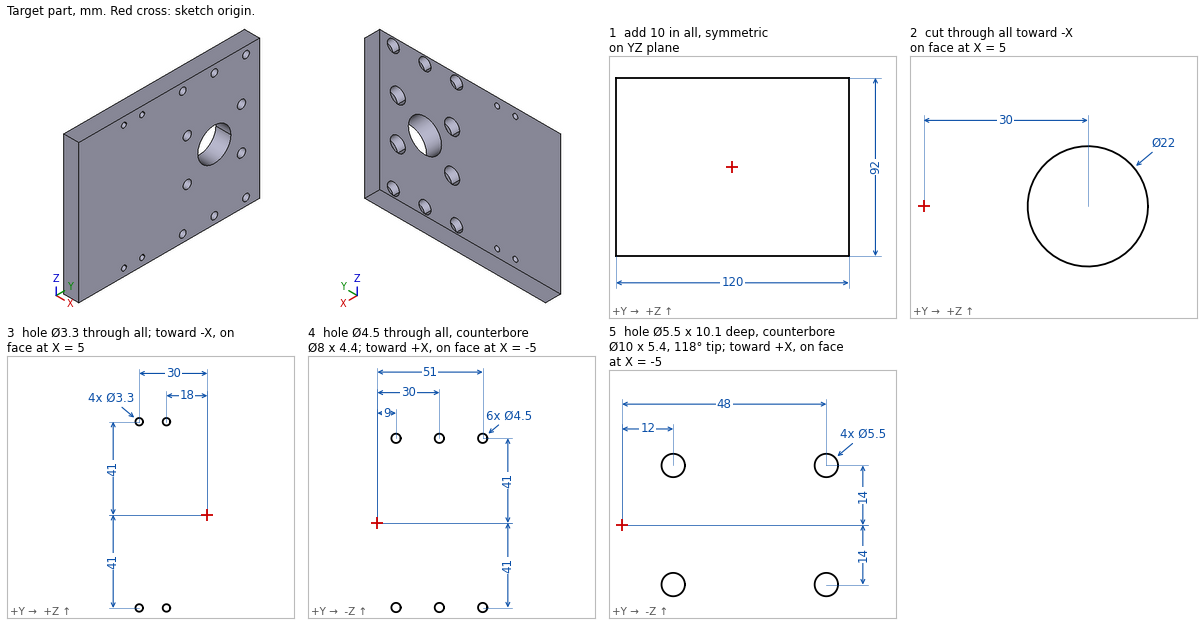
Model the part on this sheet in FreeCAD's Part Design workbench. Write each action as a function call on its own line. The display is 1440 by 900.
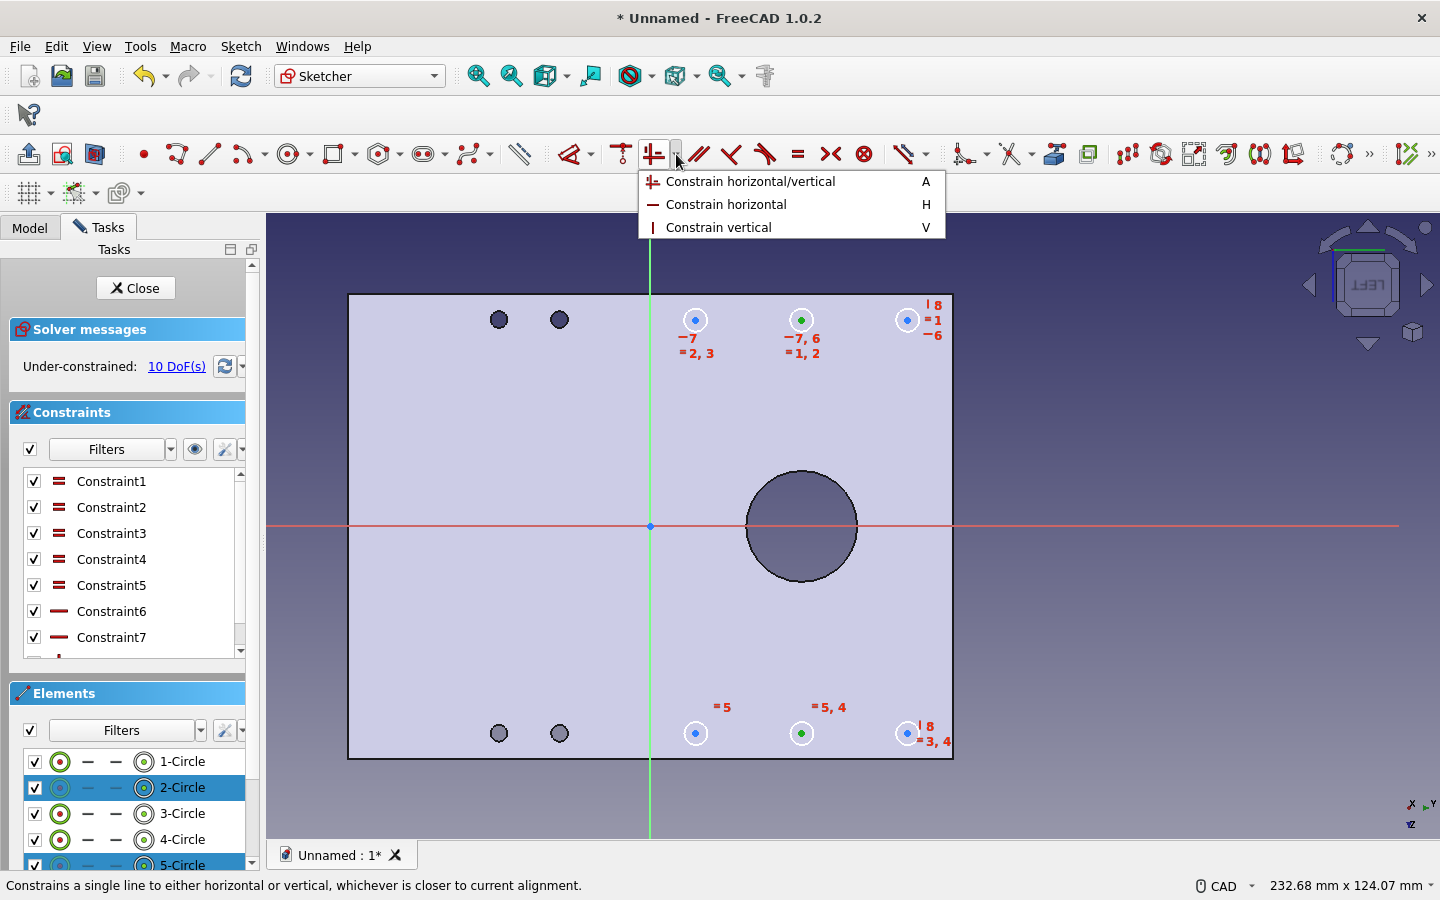
click(792, 228)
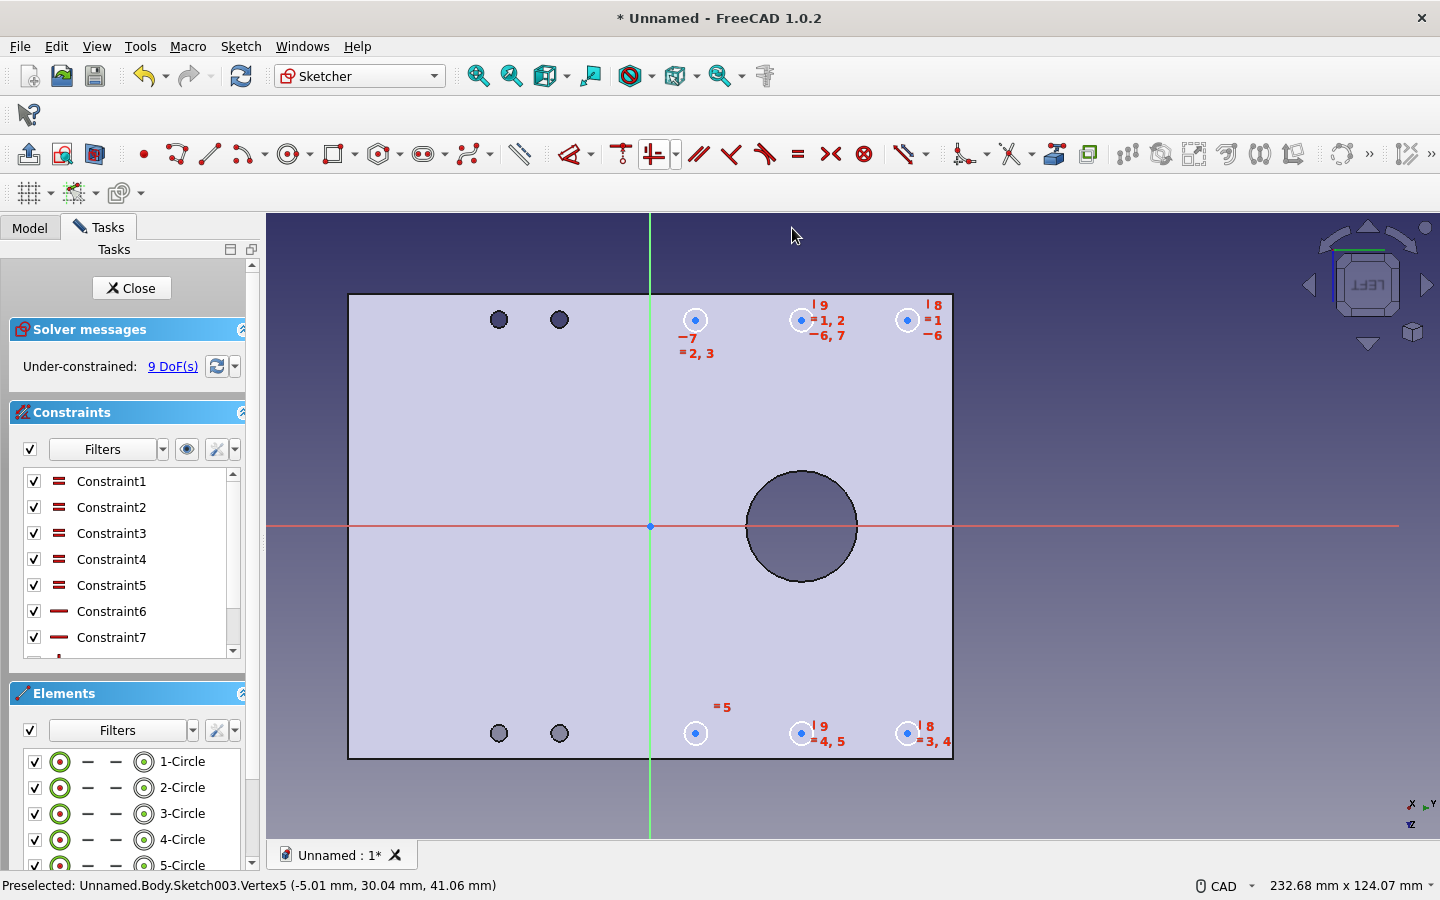
click(908, 734)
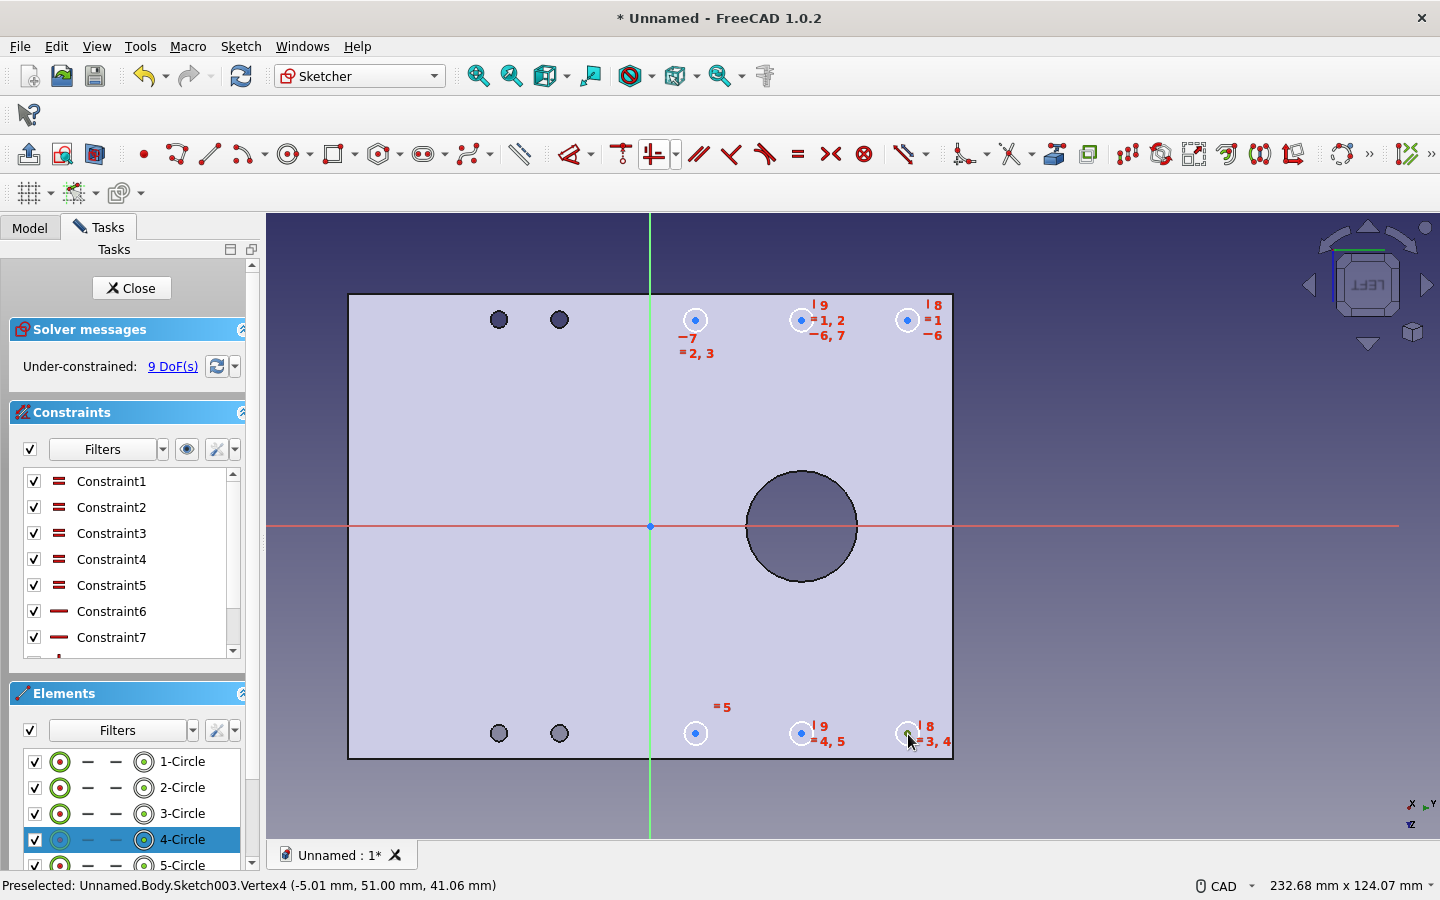
click(802, 734)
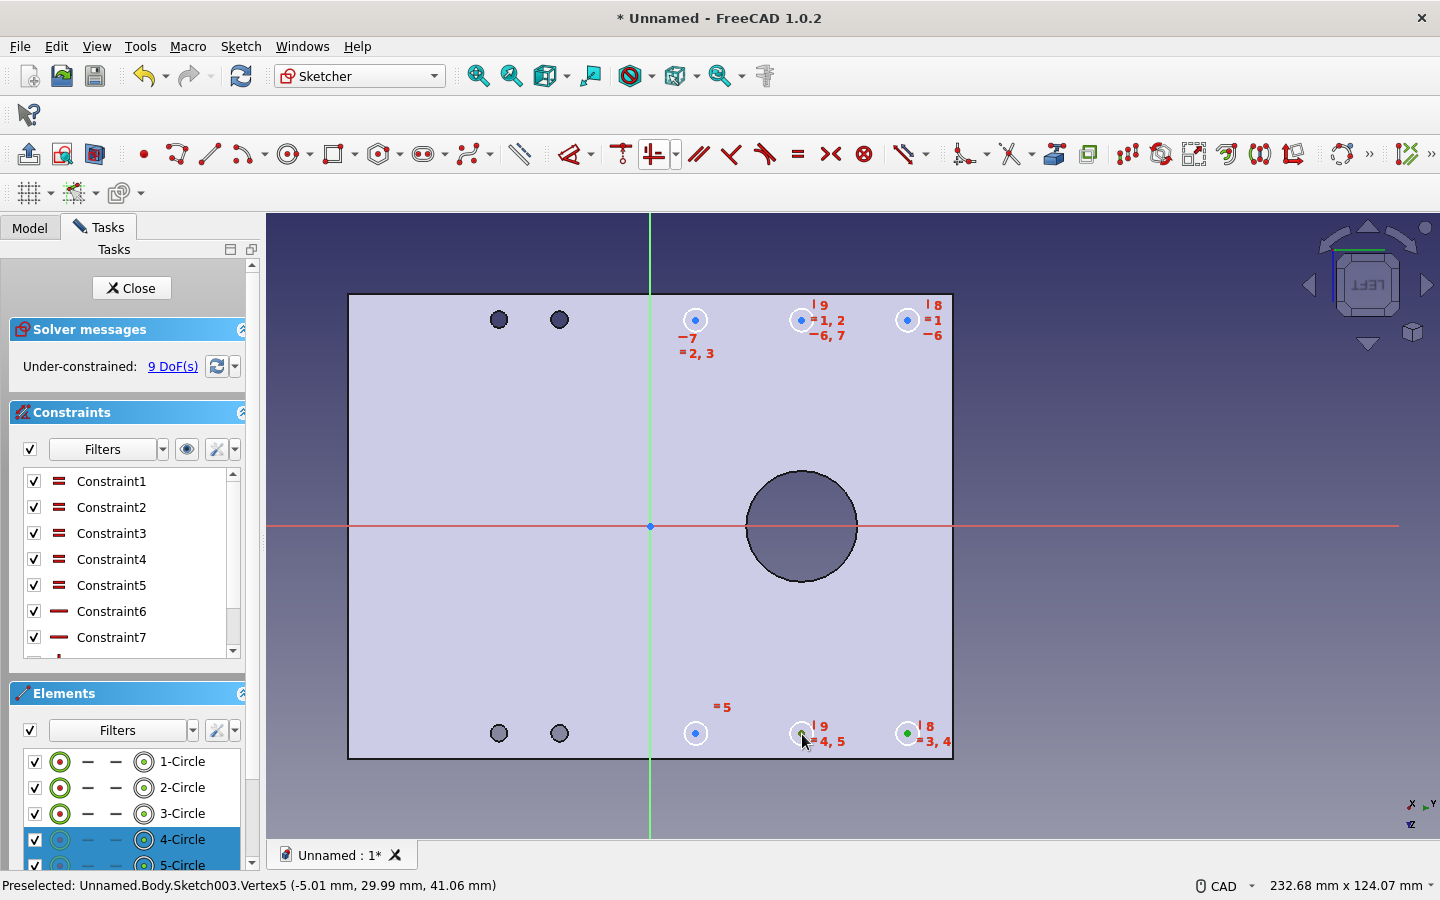
key(h)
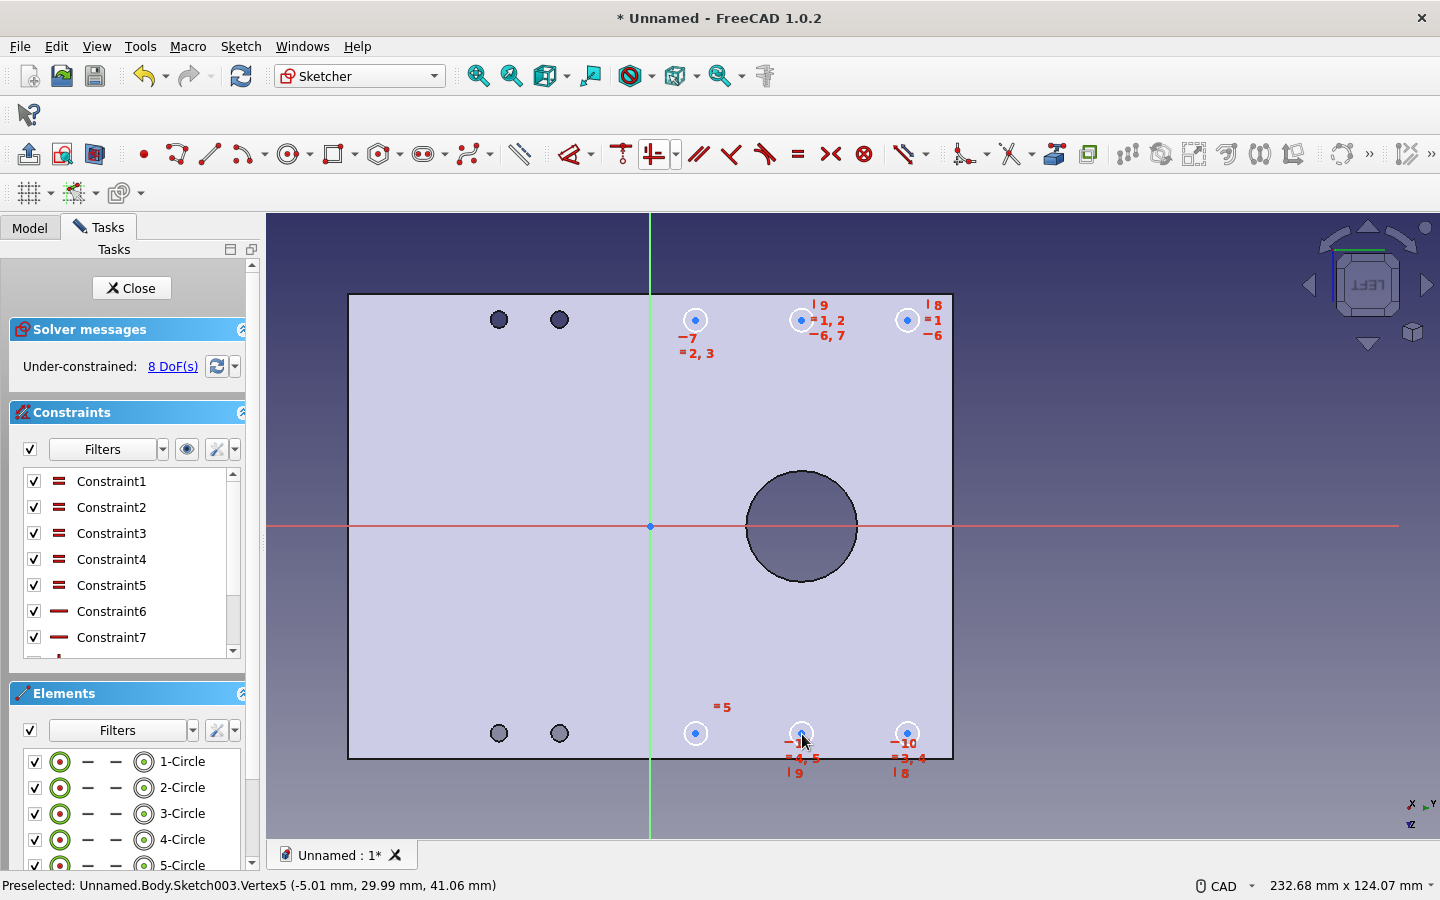
click(696, 320)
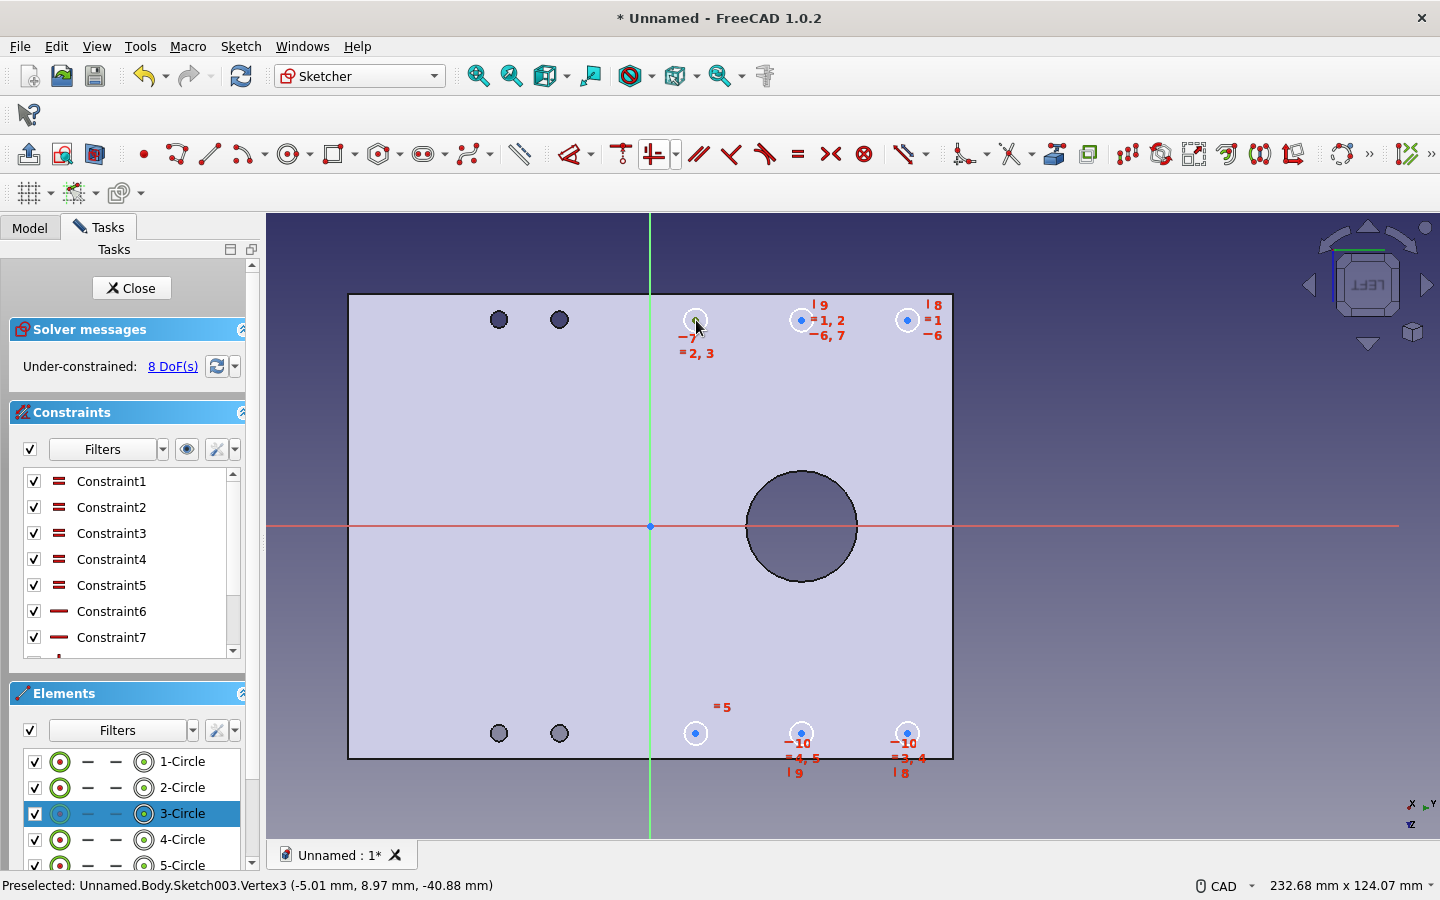
click(696, 734)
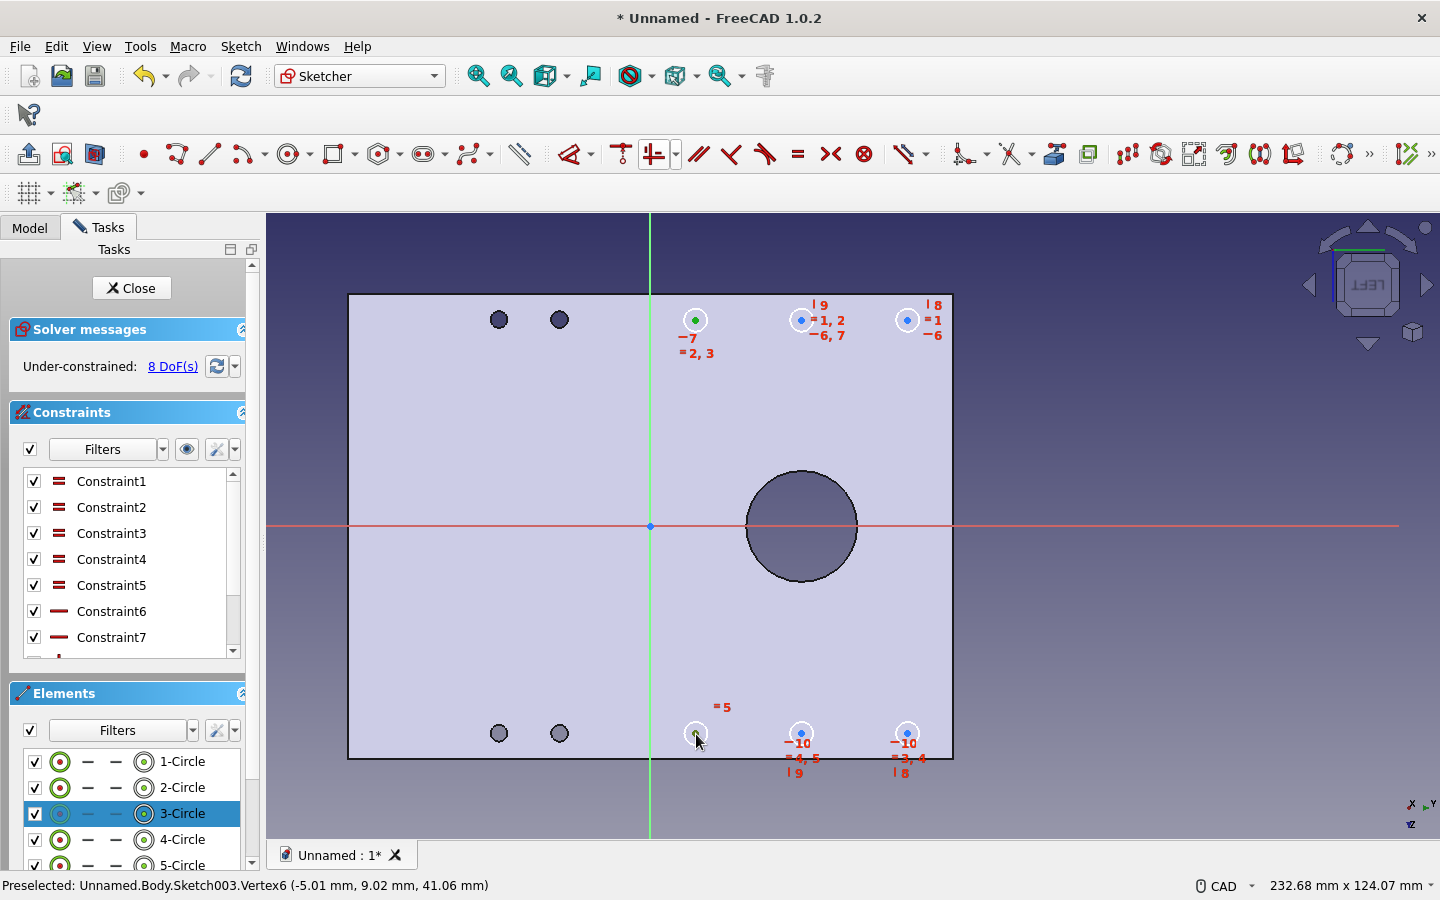
key(v)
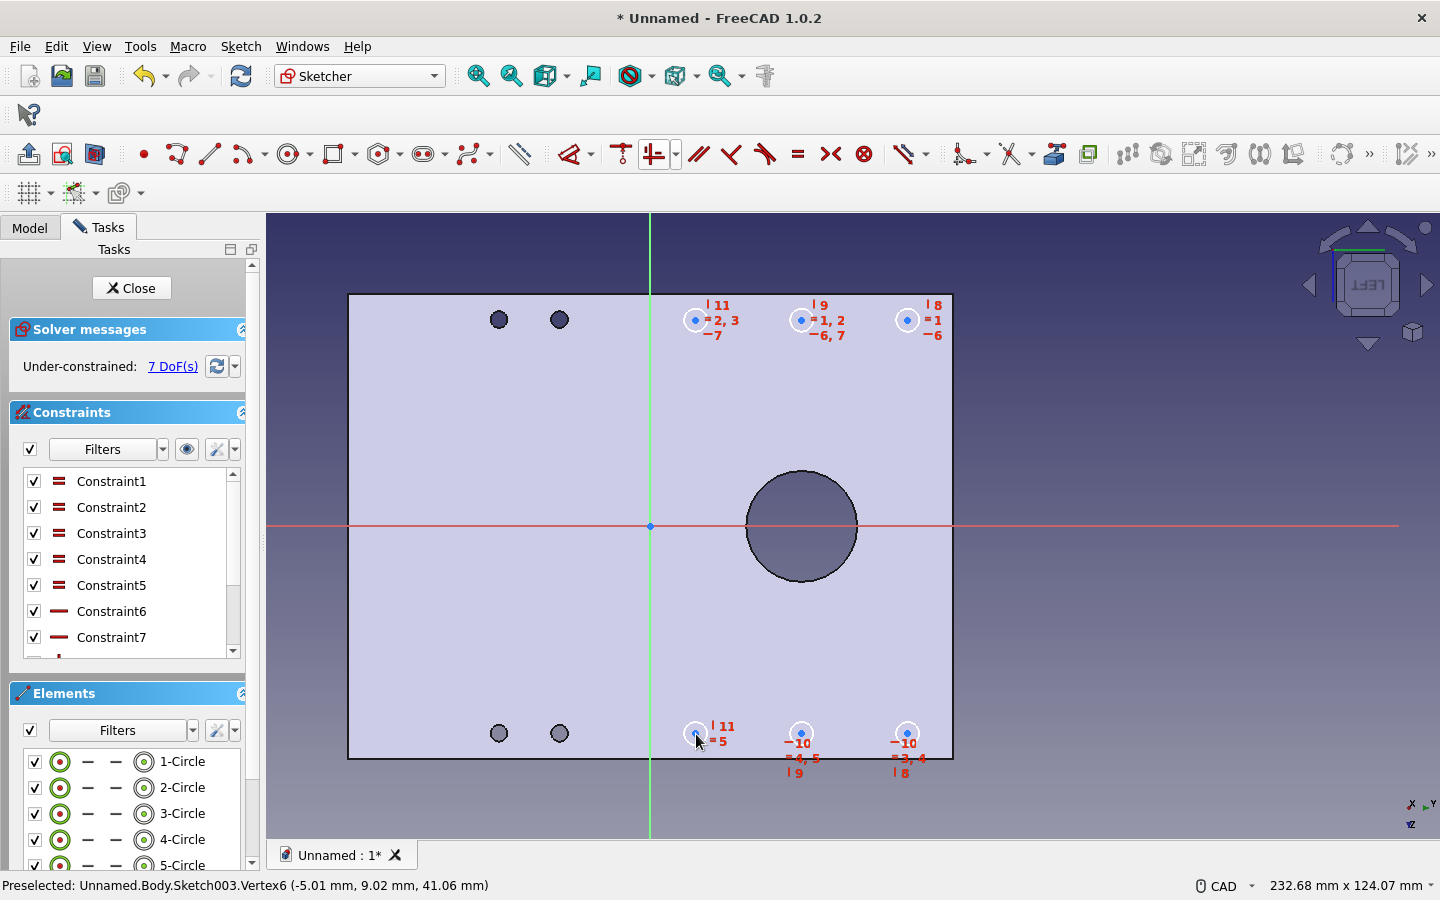
click(802, 734)